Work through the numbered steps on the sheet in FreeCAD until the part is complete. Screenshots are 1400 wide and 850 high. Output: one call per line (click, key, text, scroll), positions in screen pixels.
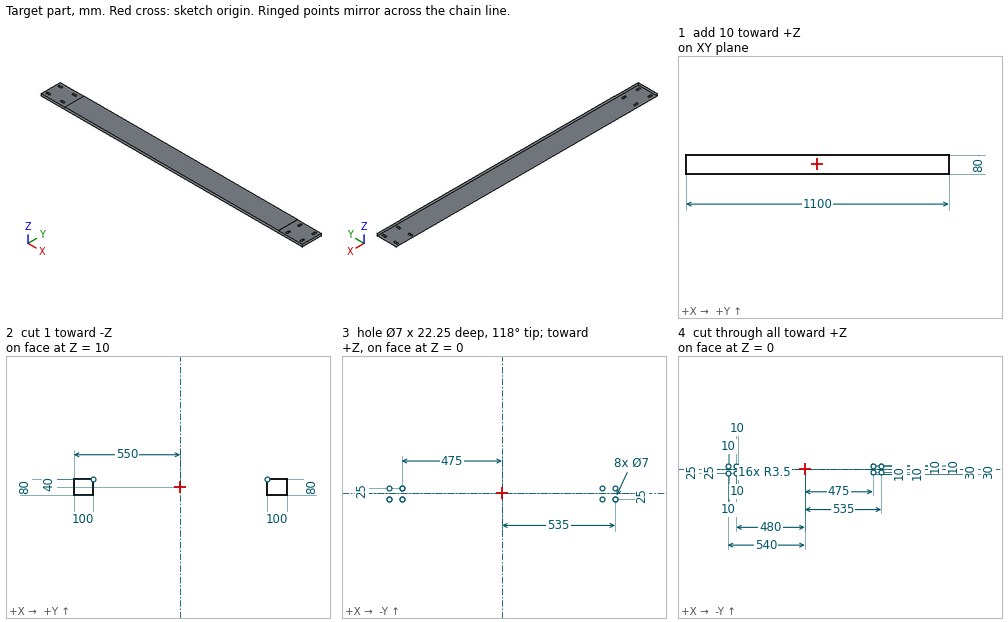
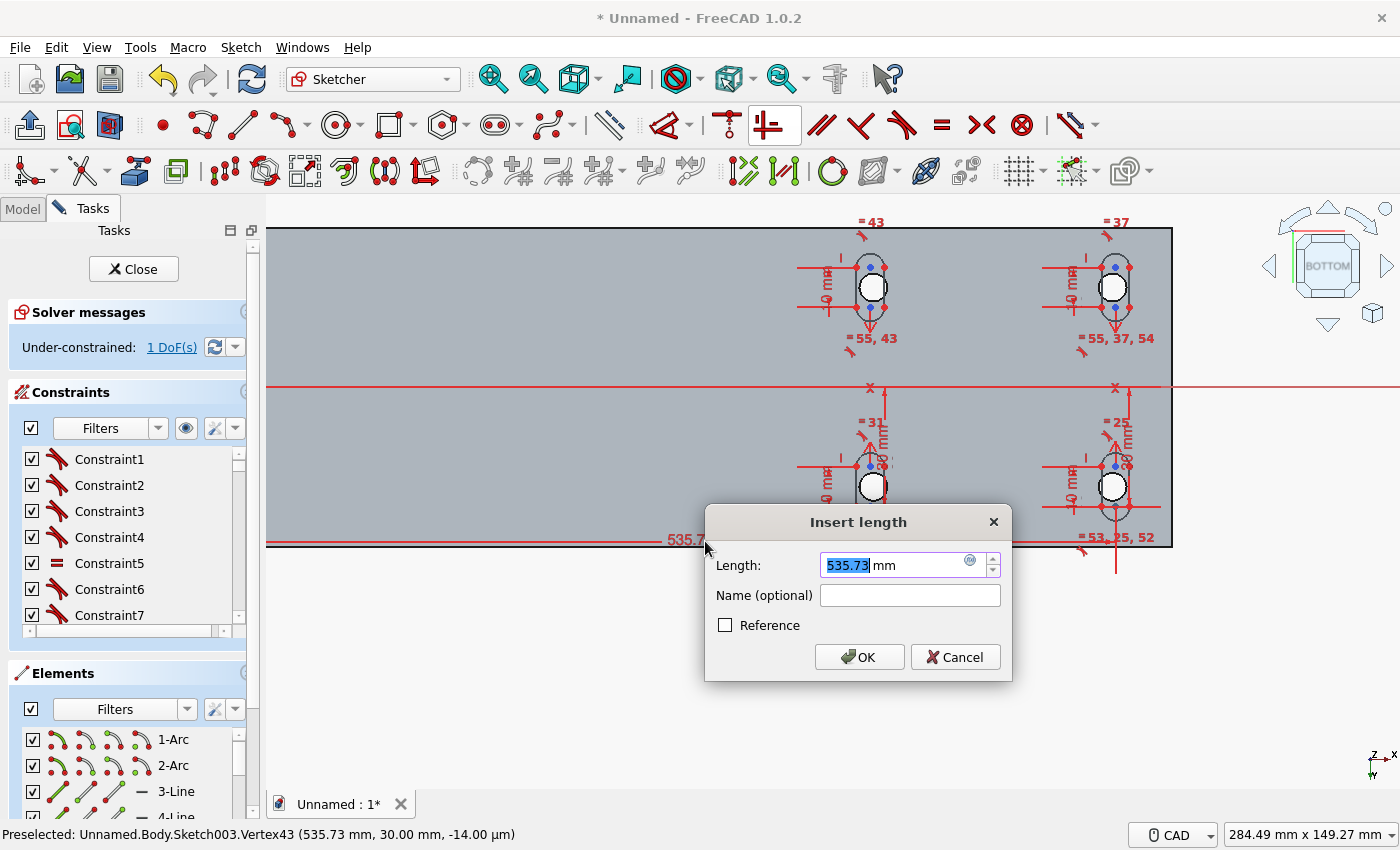
text(535)
key(Return)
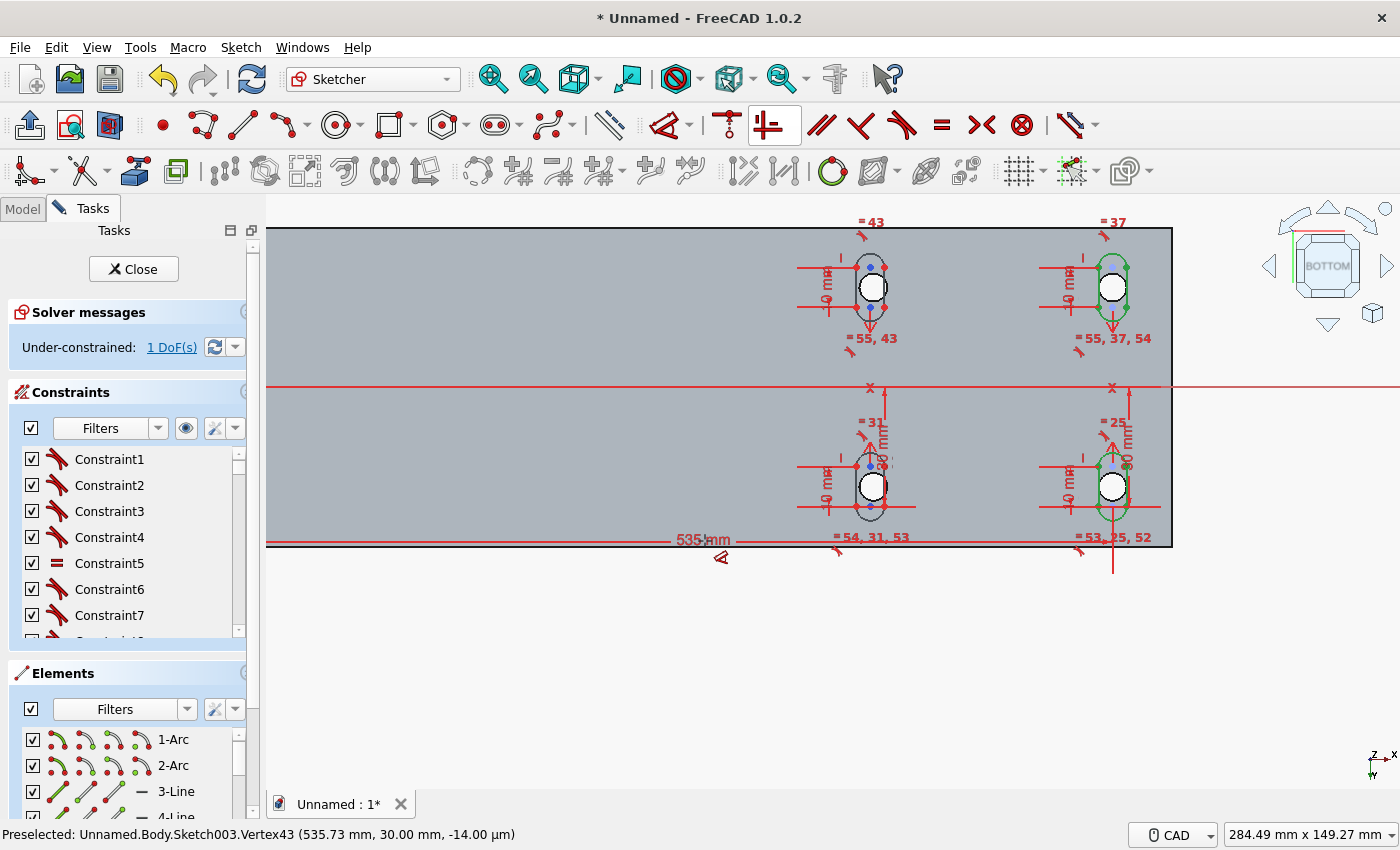
click(870, 507)
click(582, 541)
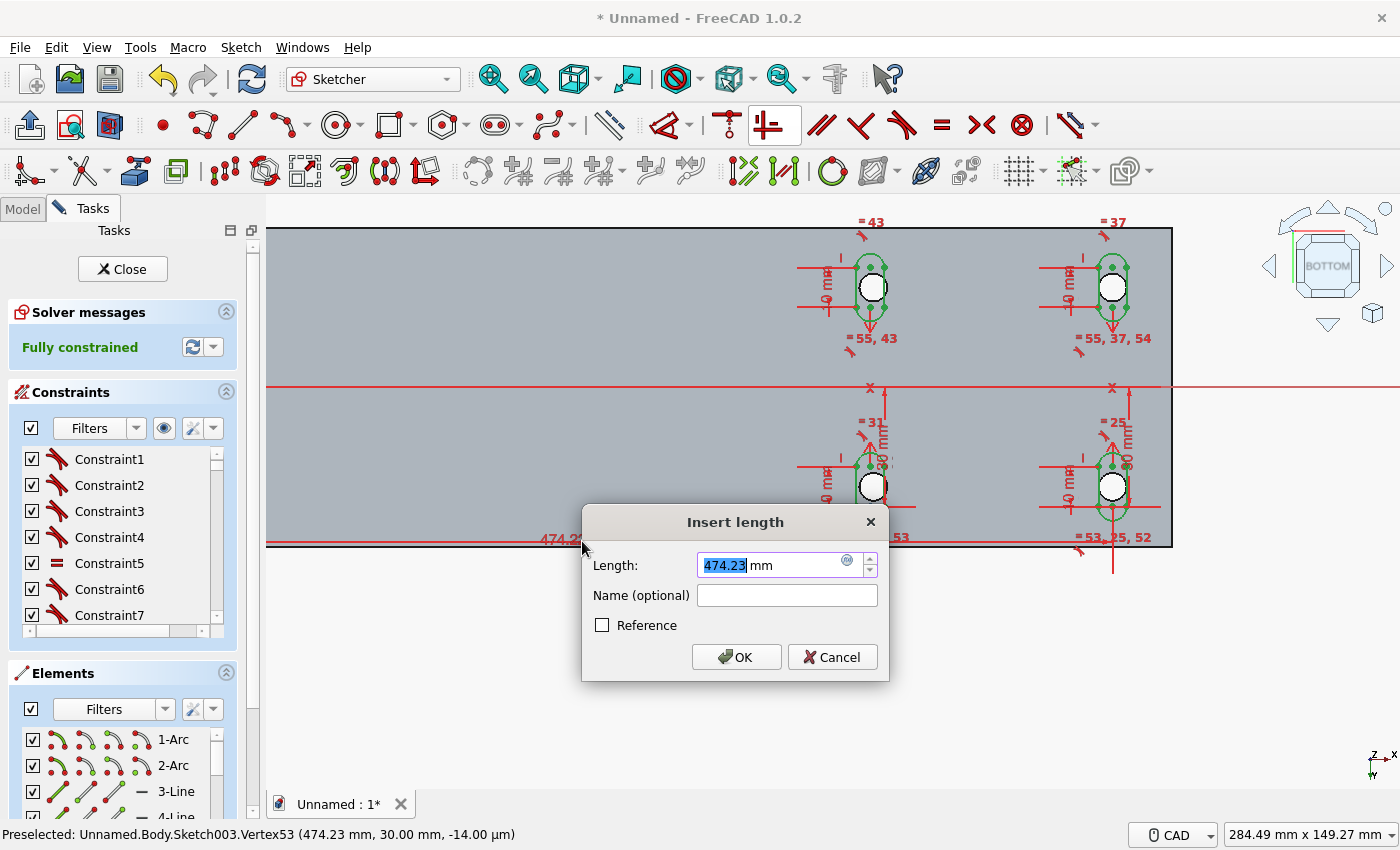
text(475)
key(Return)
key(Escape)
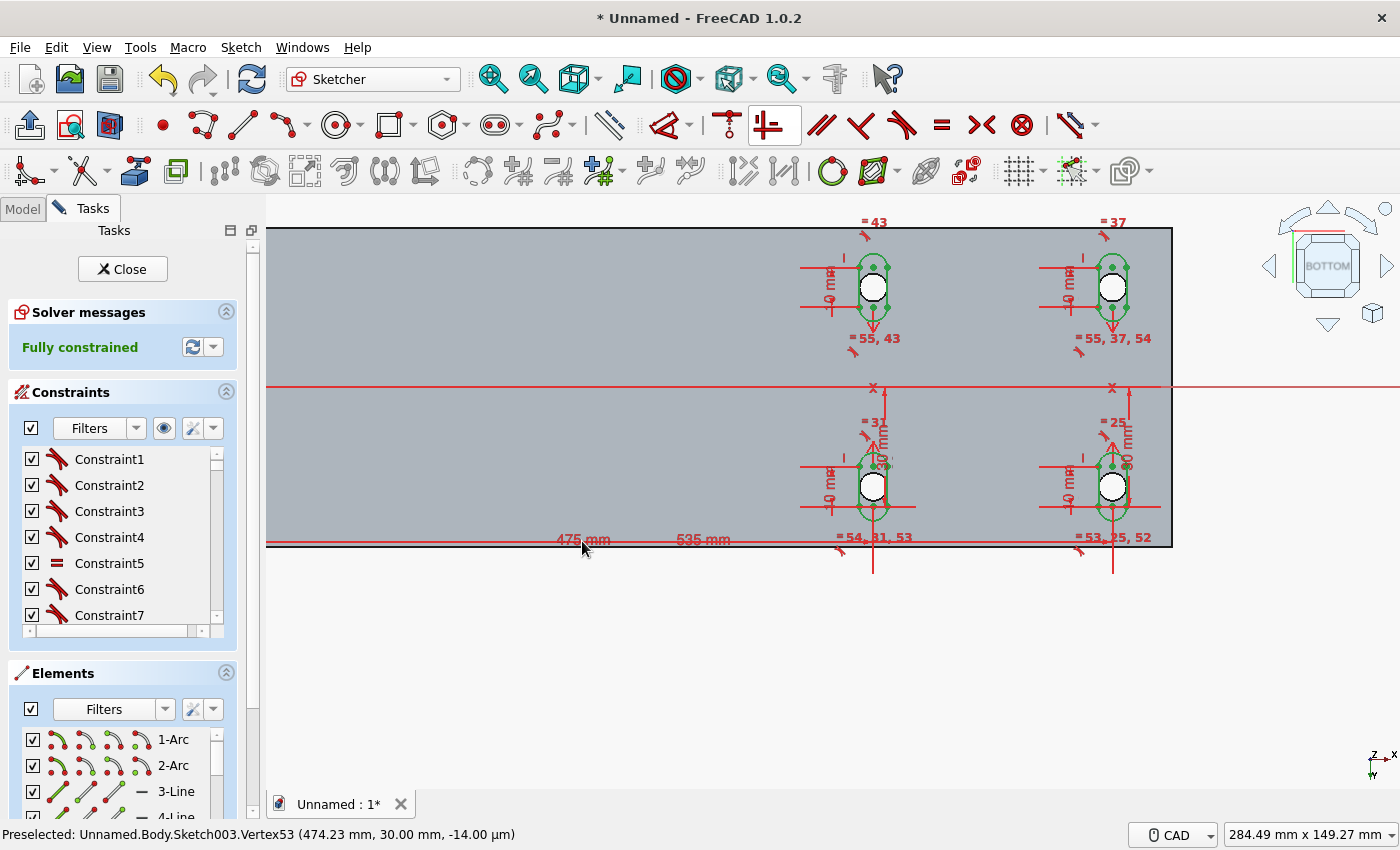
click(123, 269)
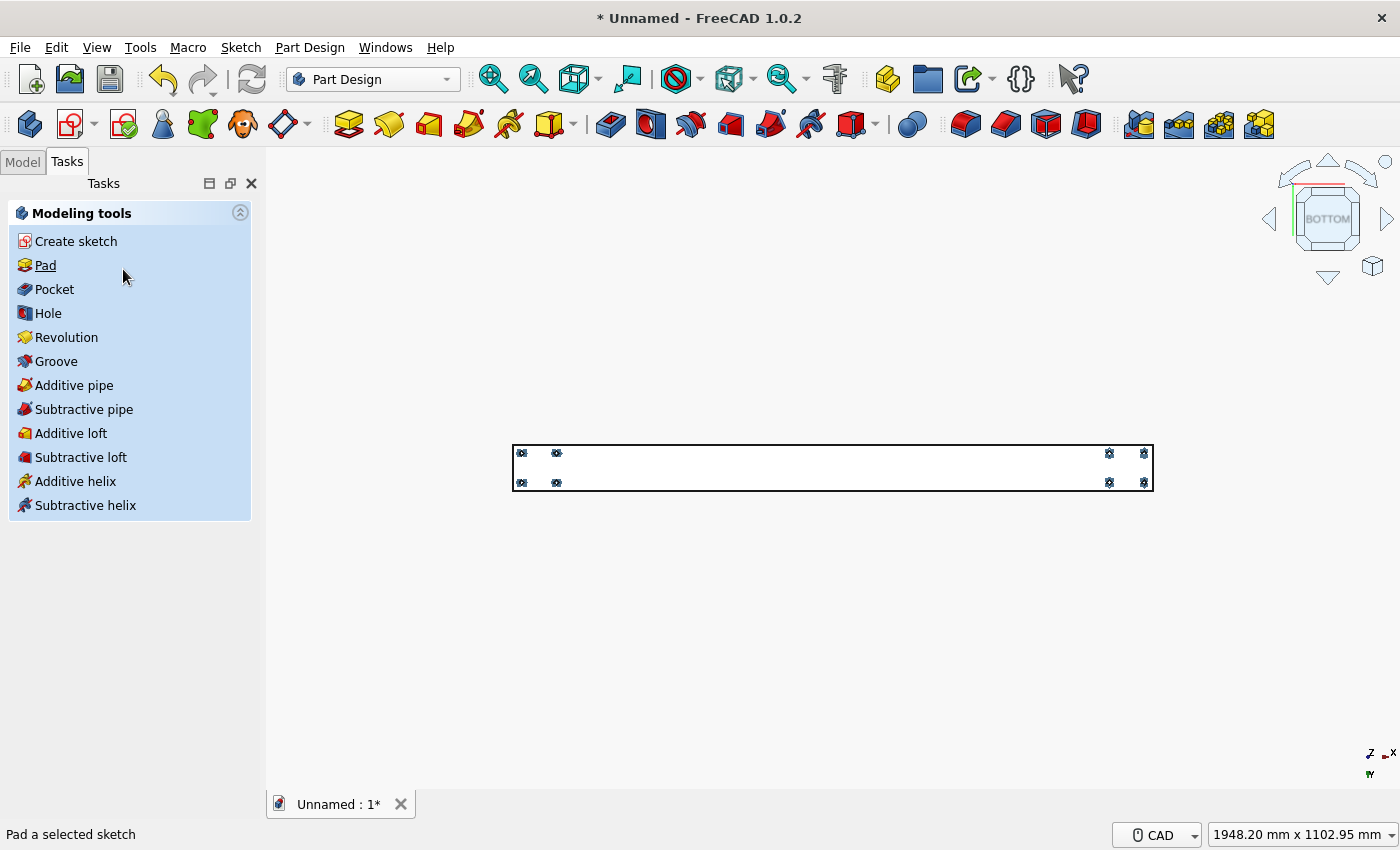
click(612, 124)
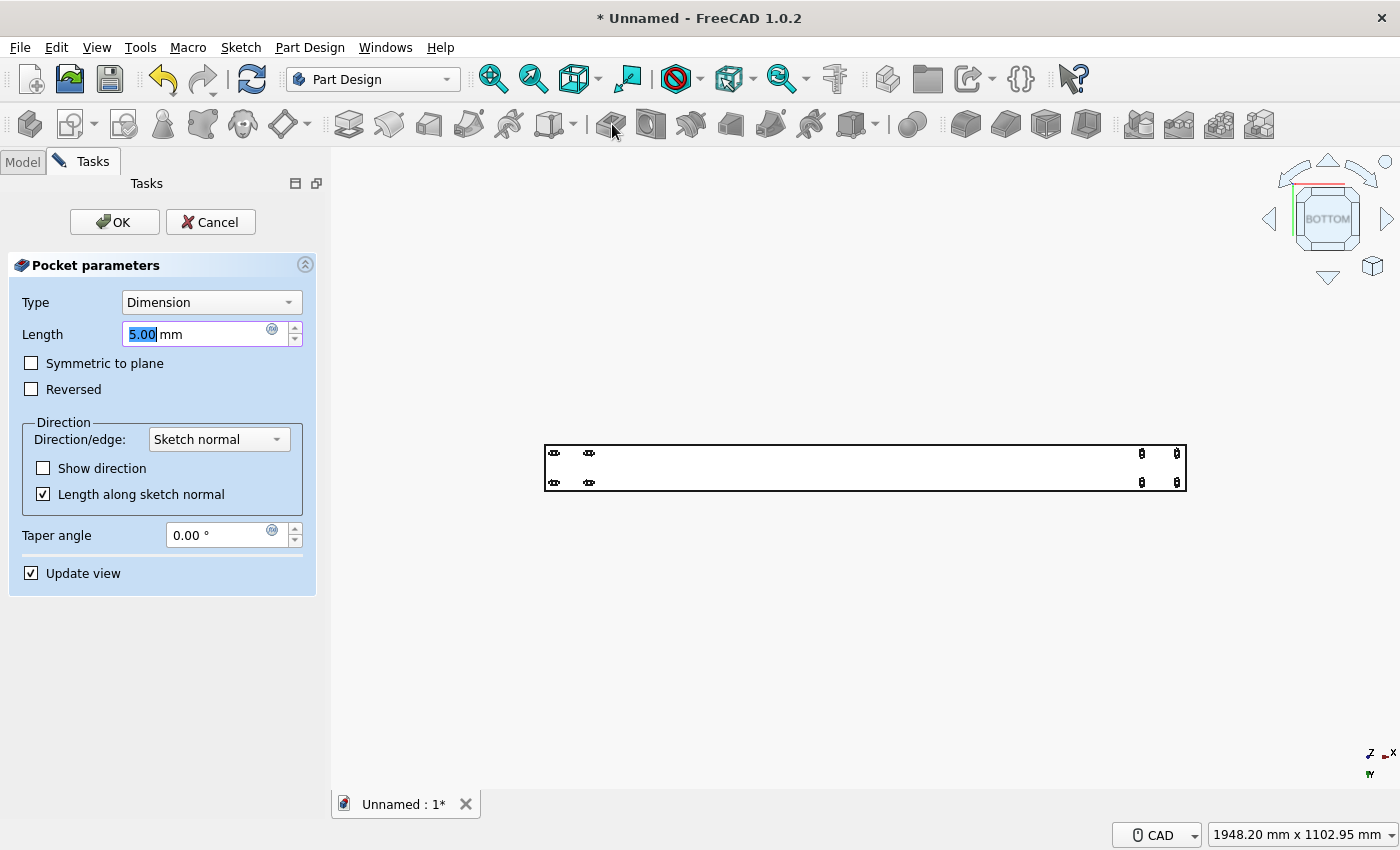
click(212, 302)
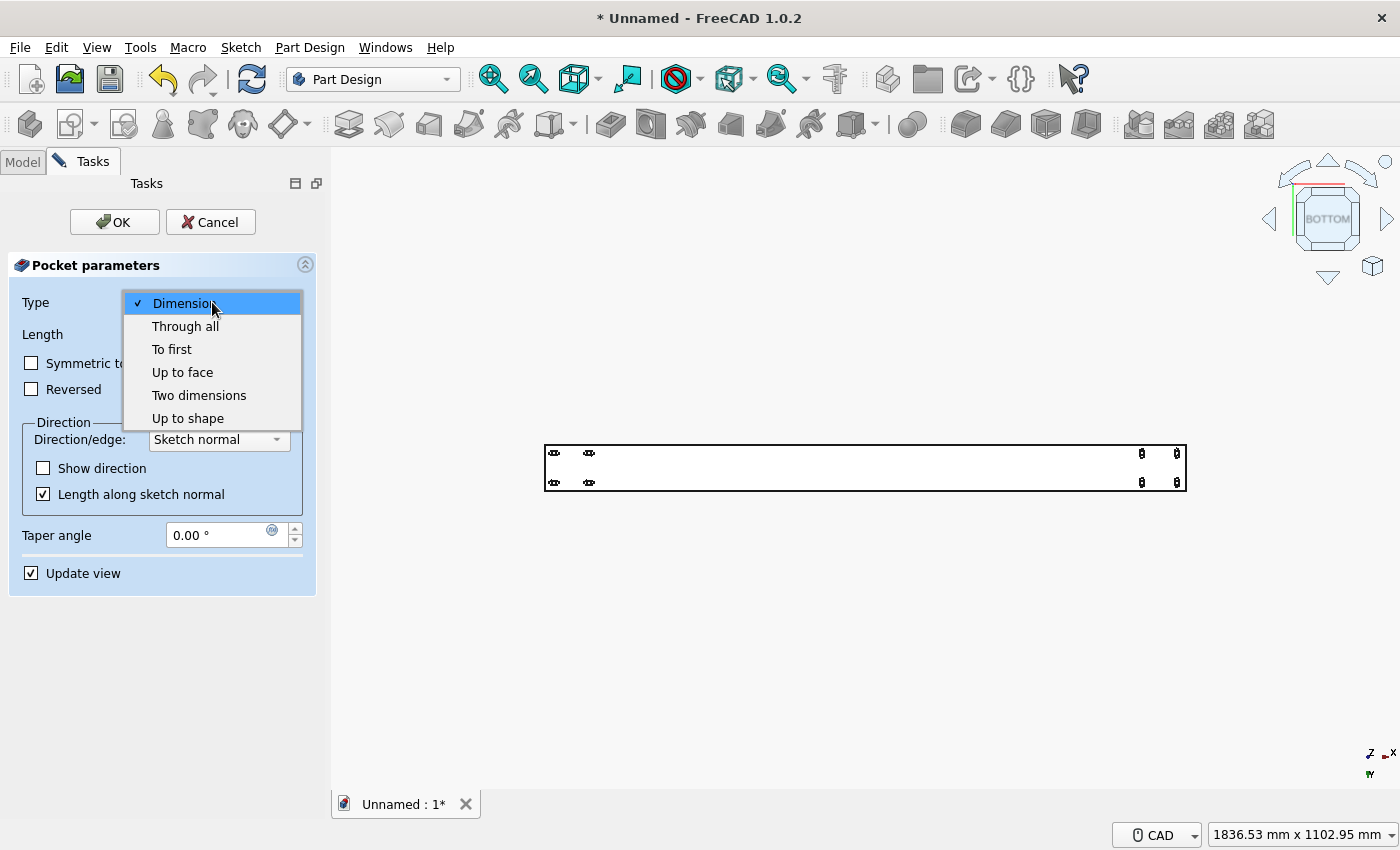
click(212, 326)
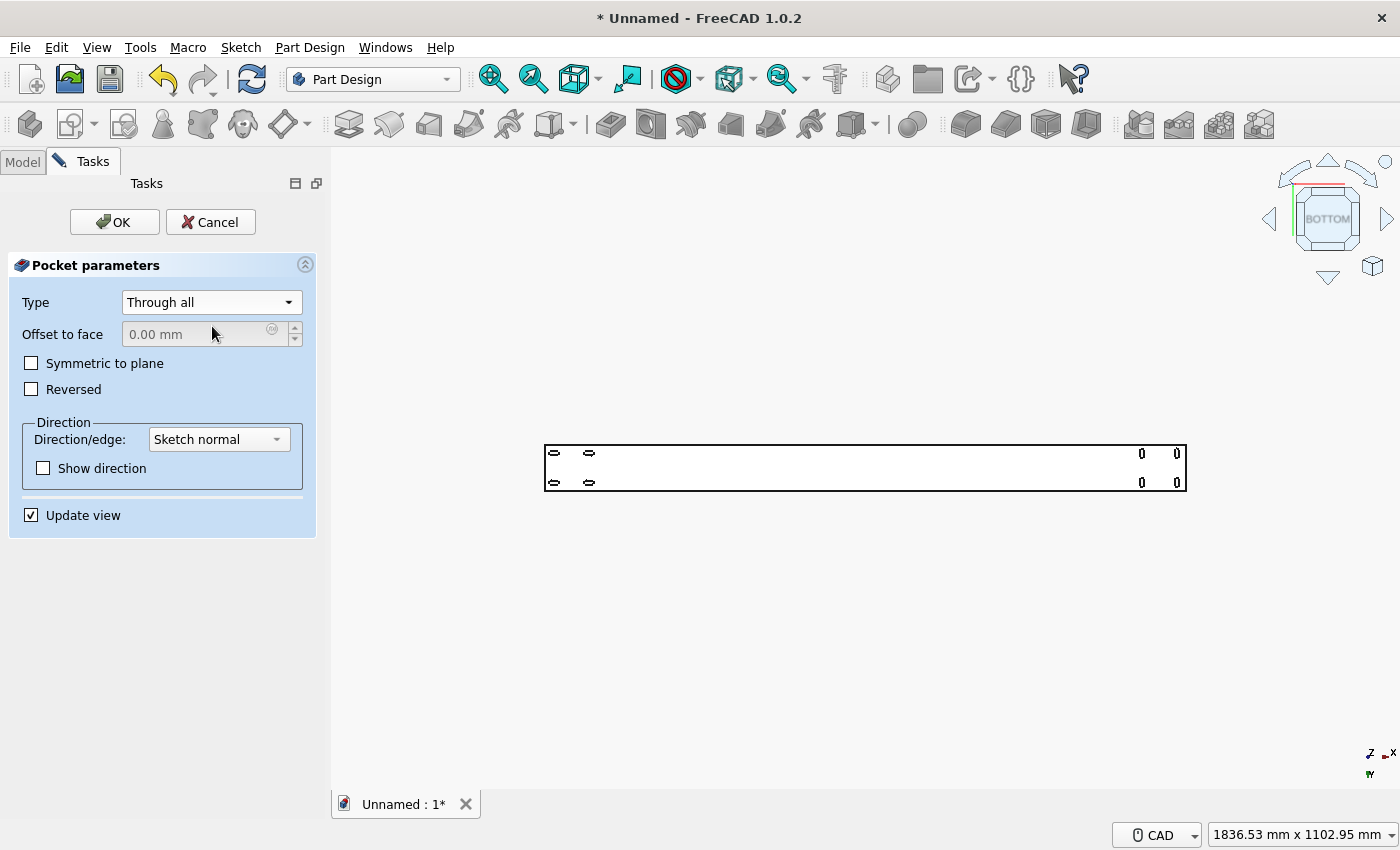
click(115, 222)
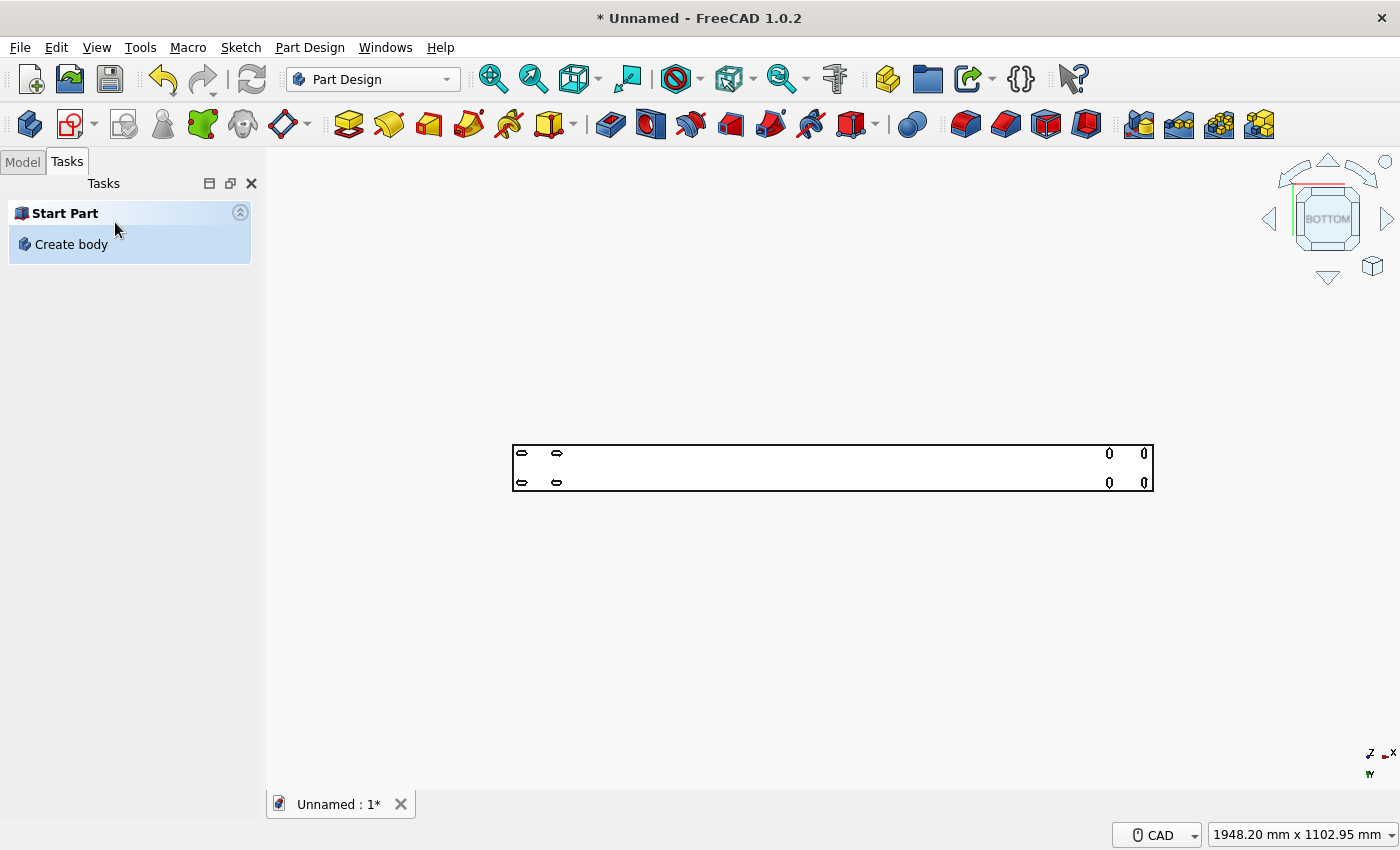
key(0)